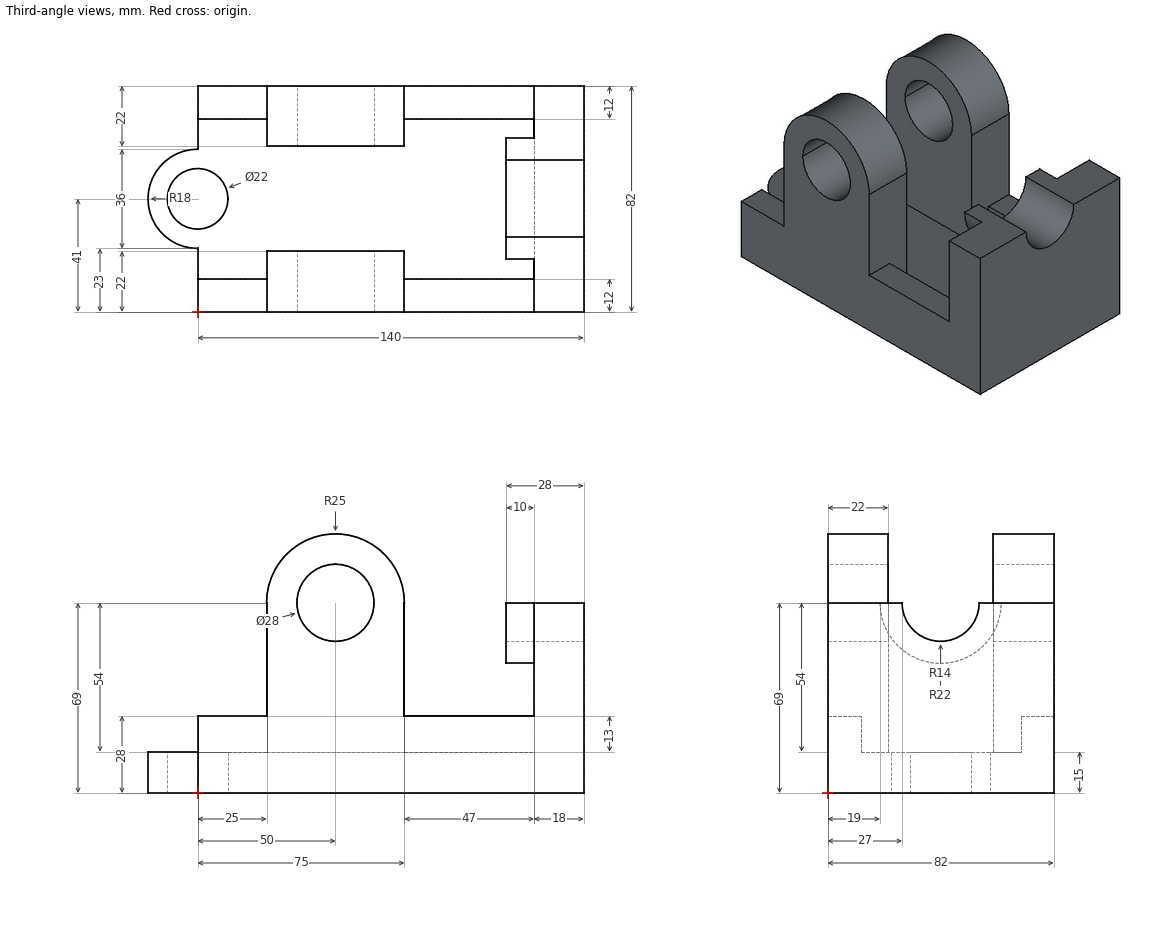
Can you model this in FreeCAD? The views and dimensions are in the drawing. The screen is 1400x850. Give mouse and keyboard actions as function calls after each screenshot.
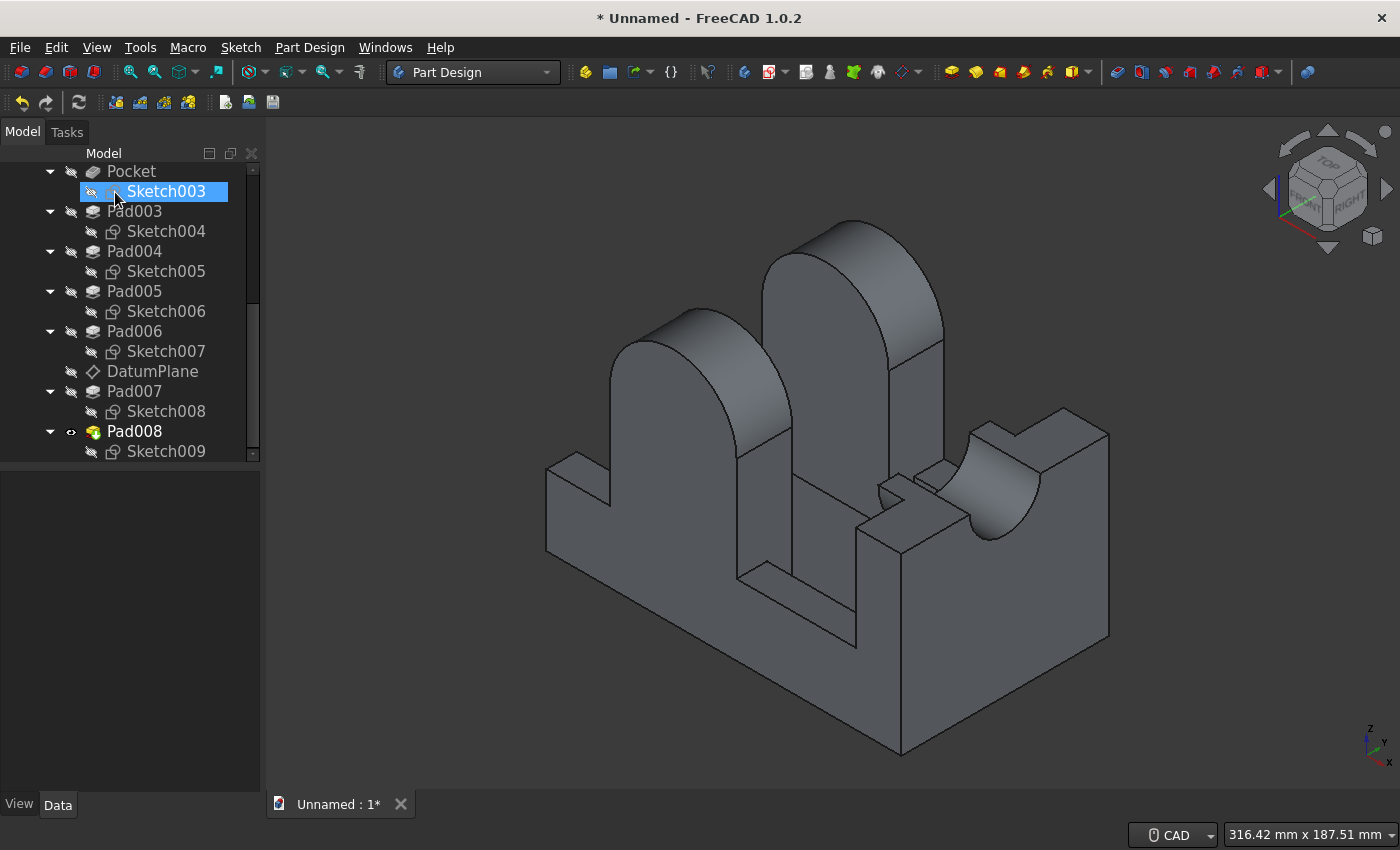
click(805, 535)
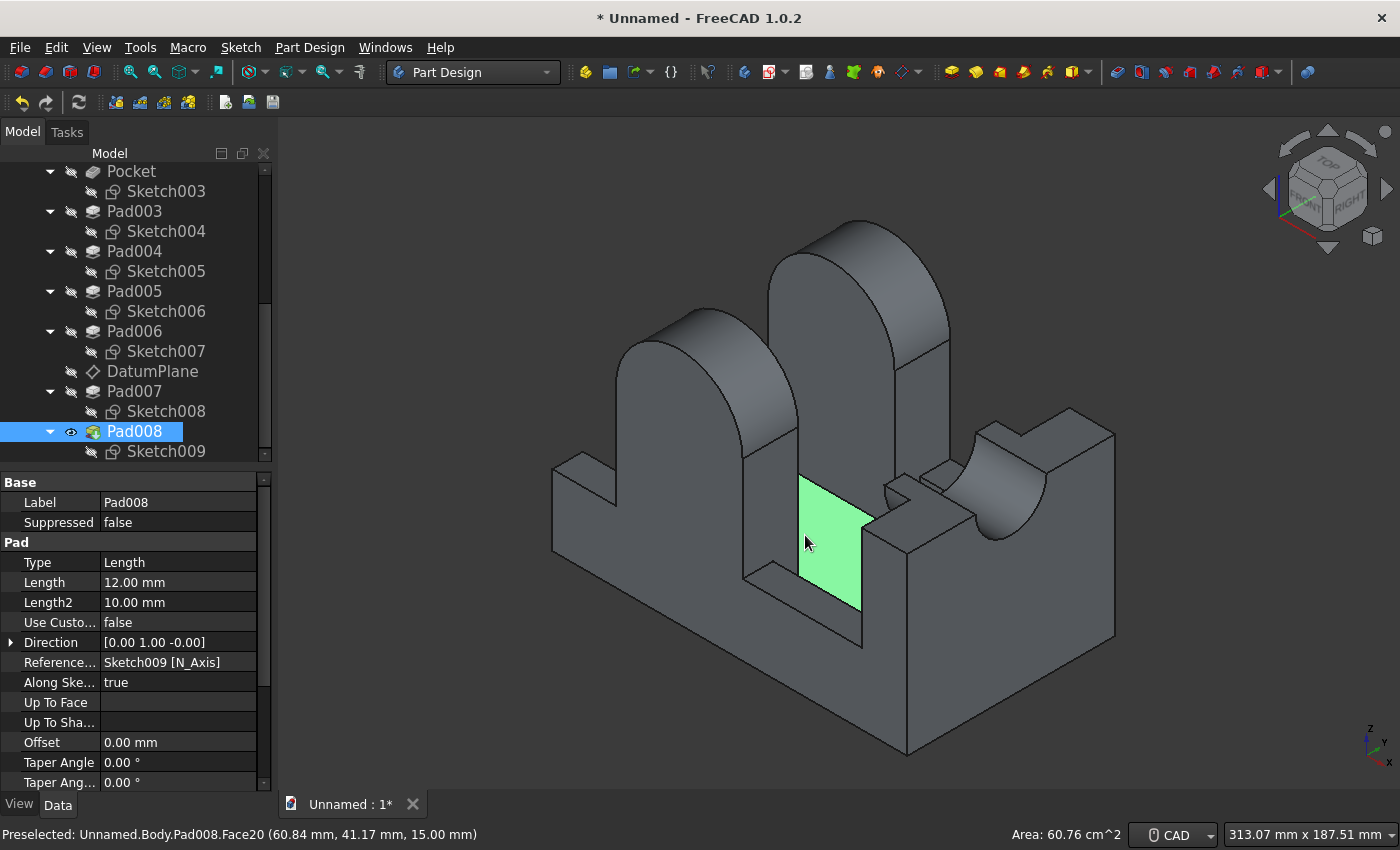
click(770, 72)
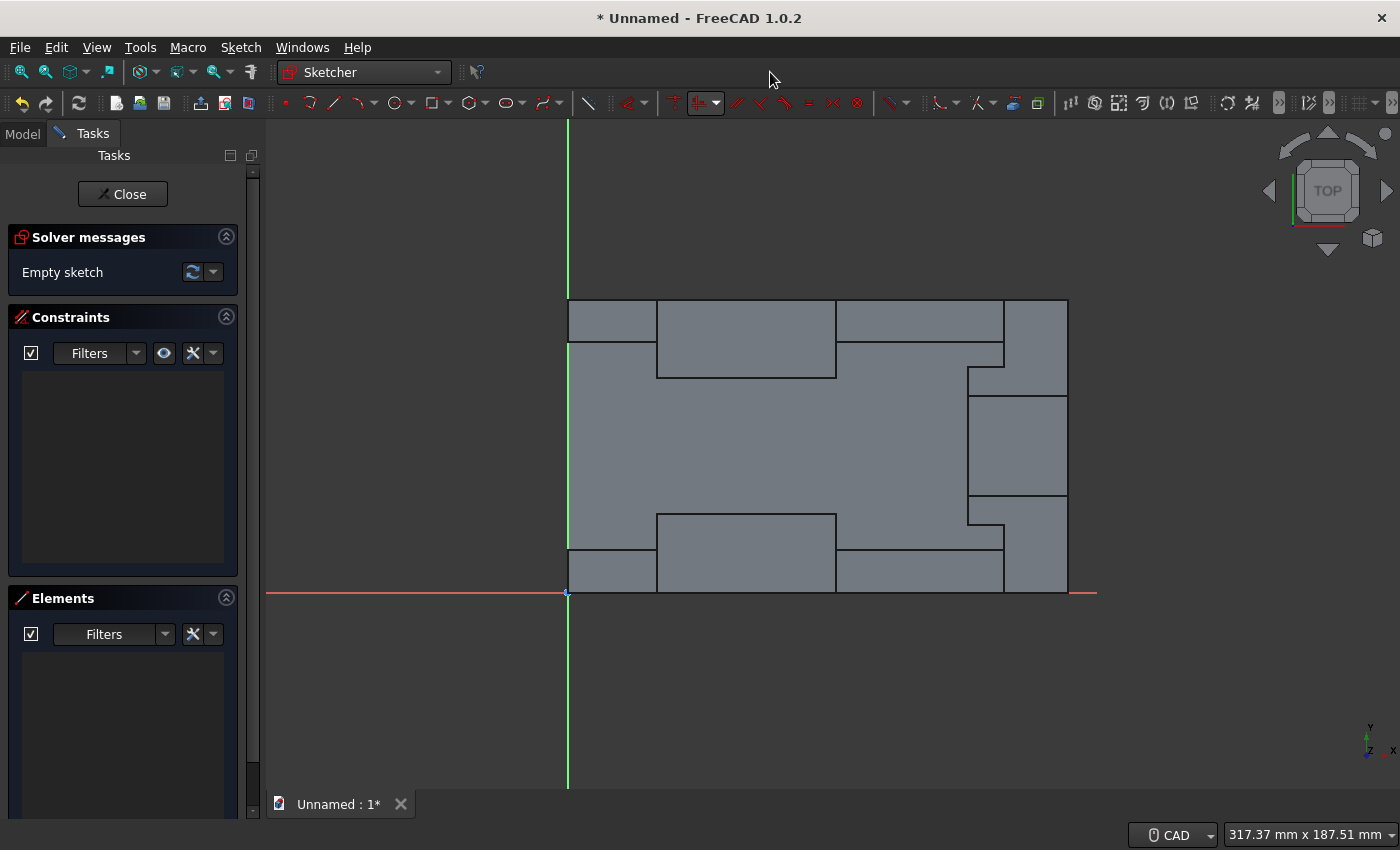
scroll(349, 514, up, 4)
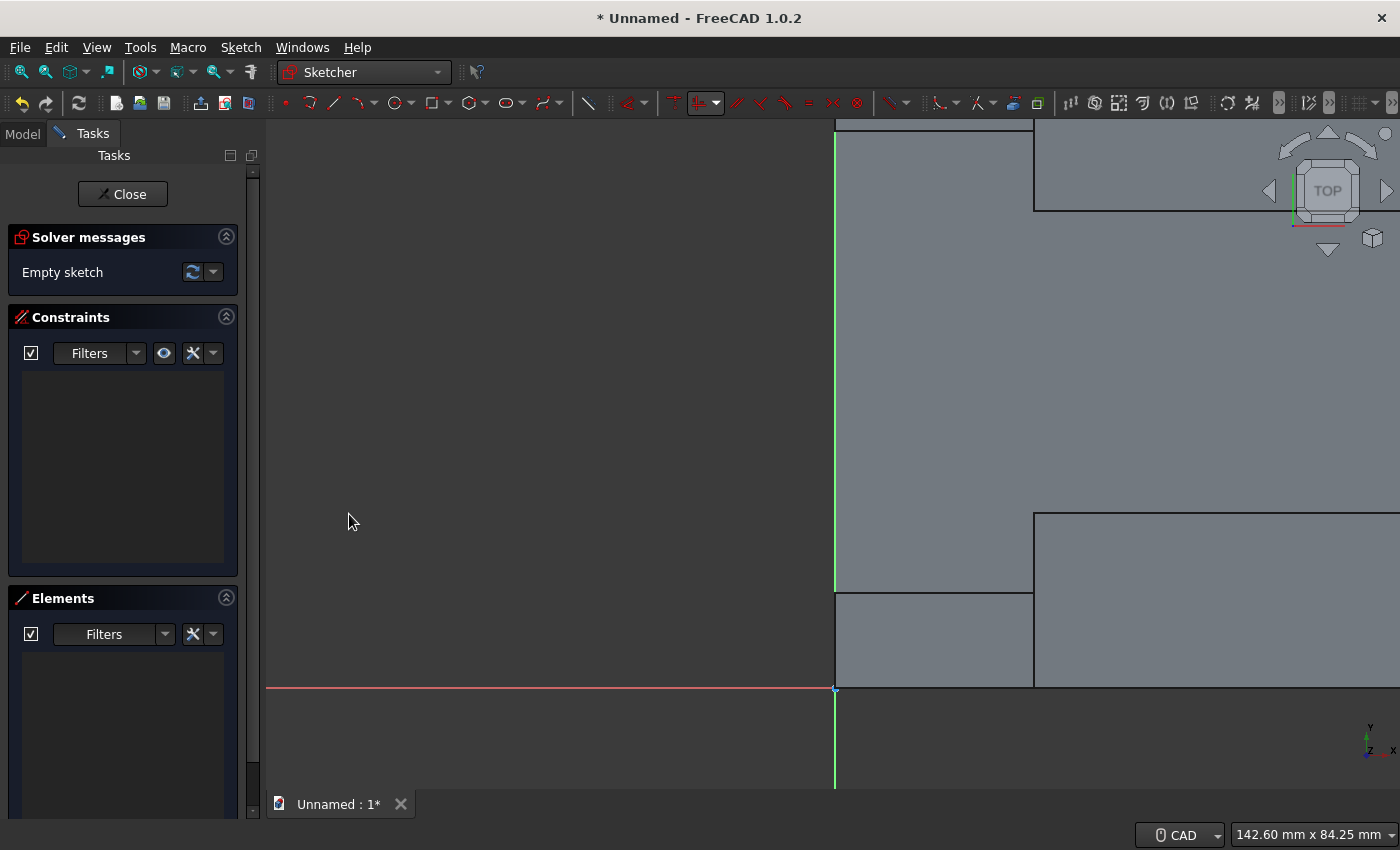
click(334, 104)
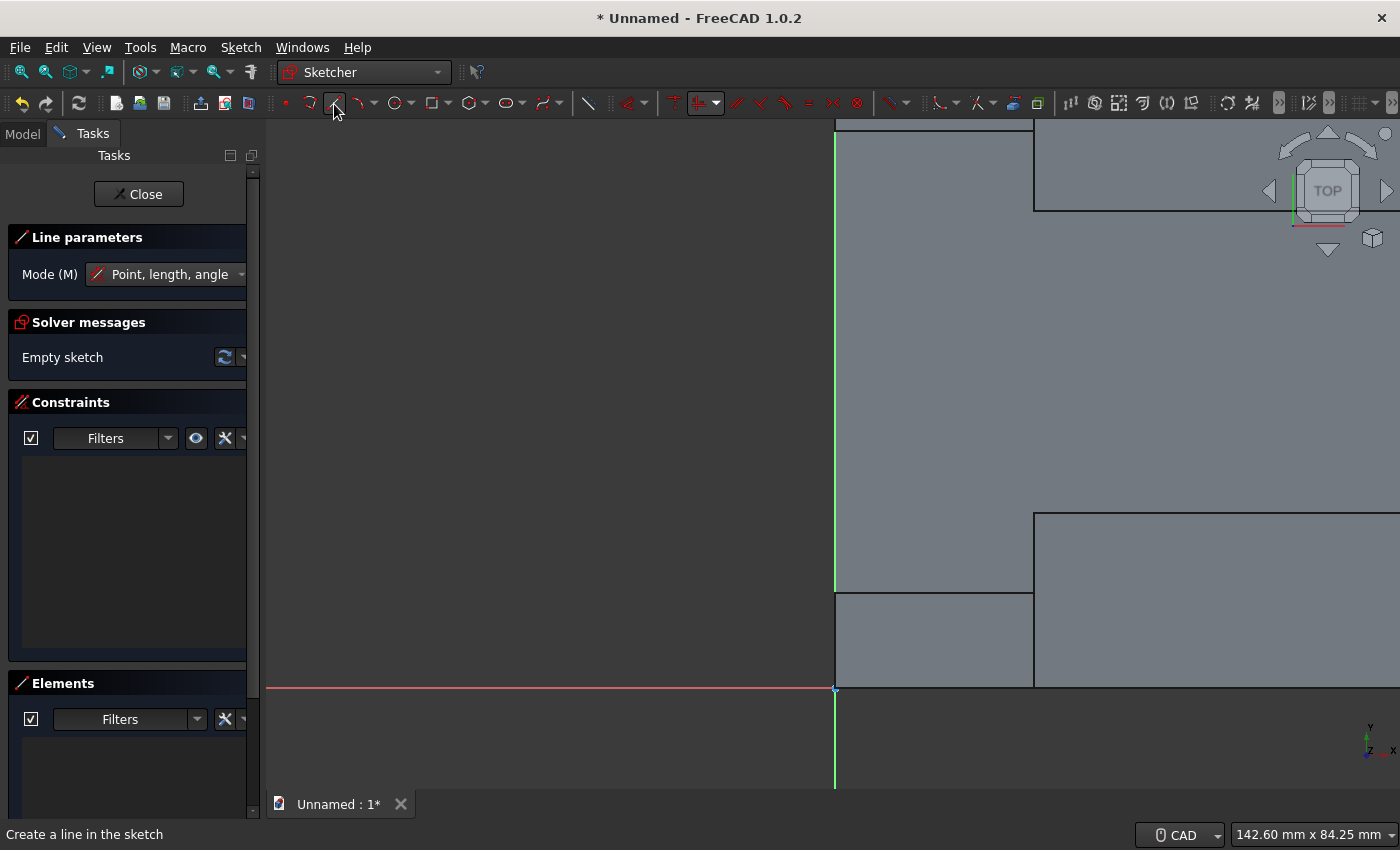
click(835, 505)
click(826, 219)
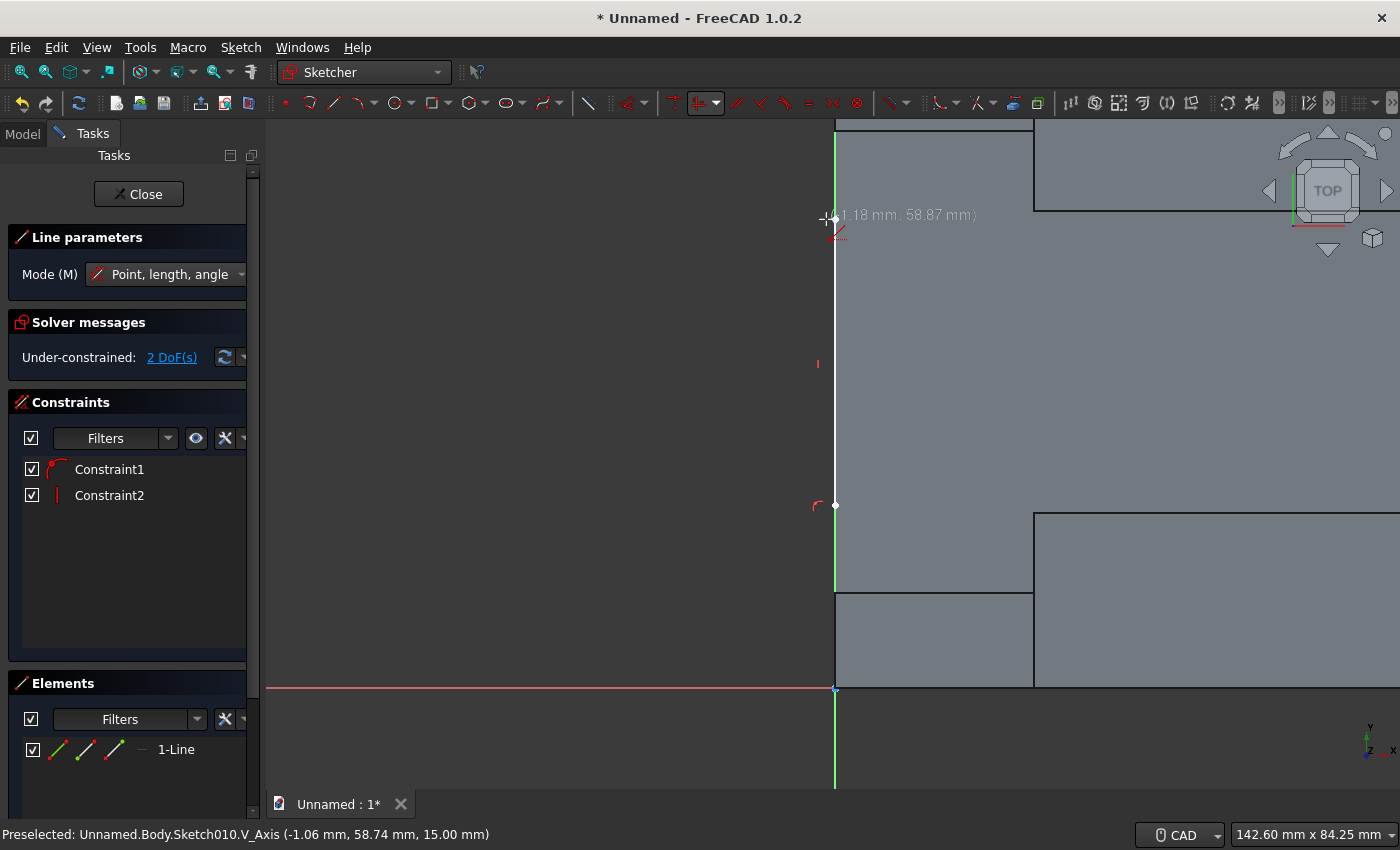
click(358, 104)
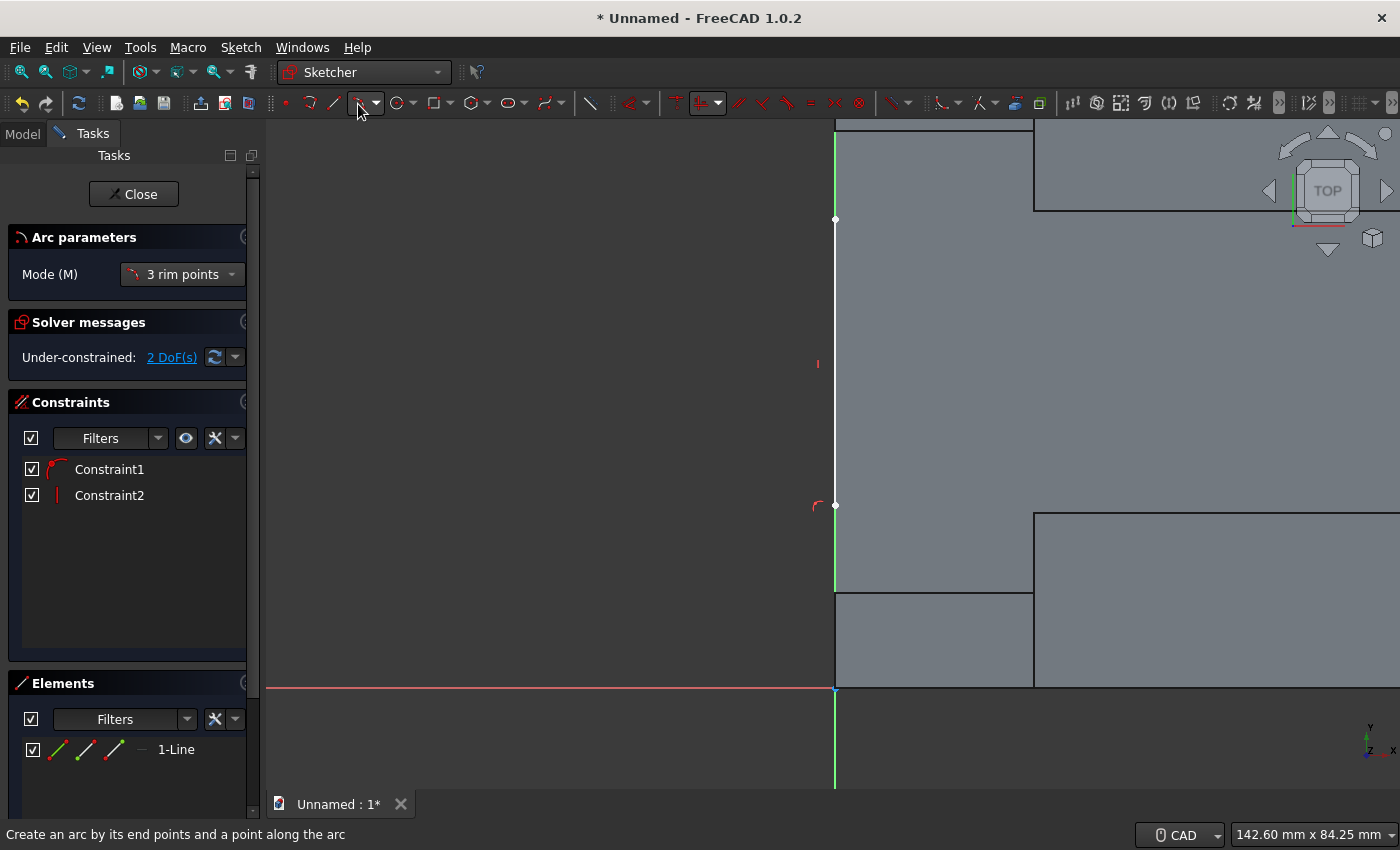
click(826, 219)
click(835, 506)
click(692, 362)
key(Escape)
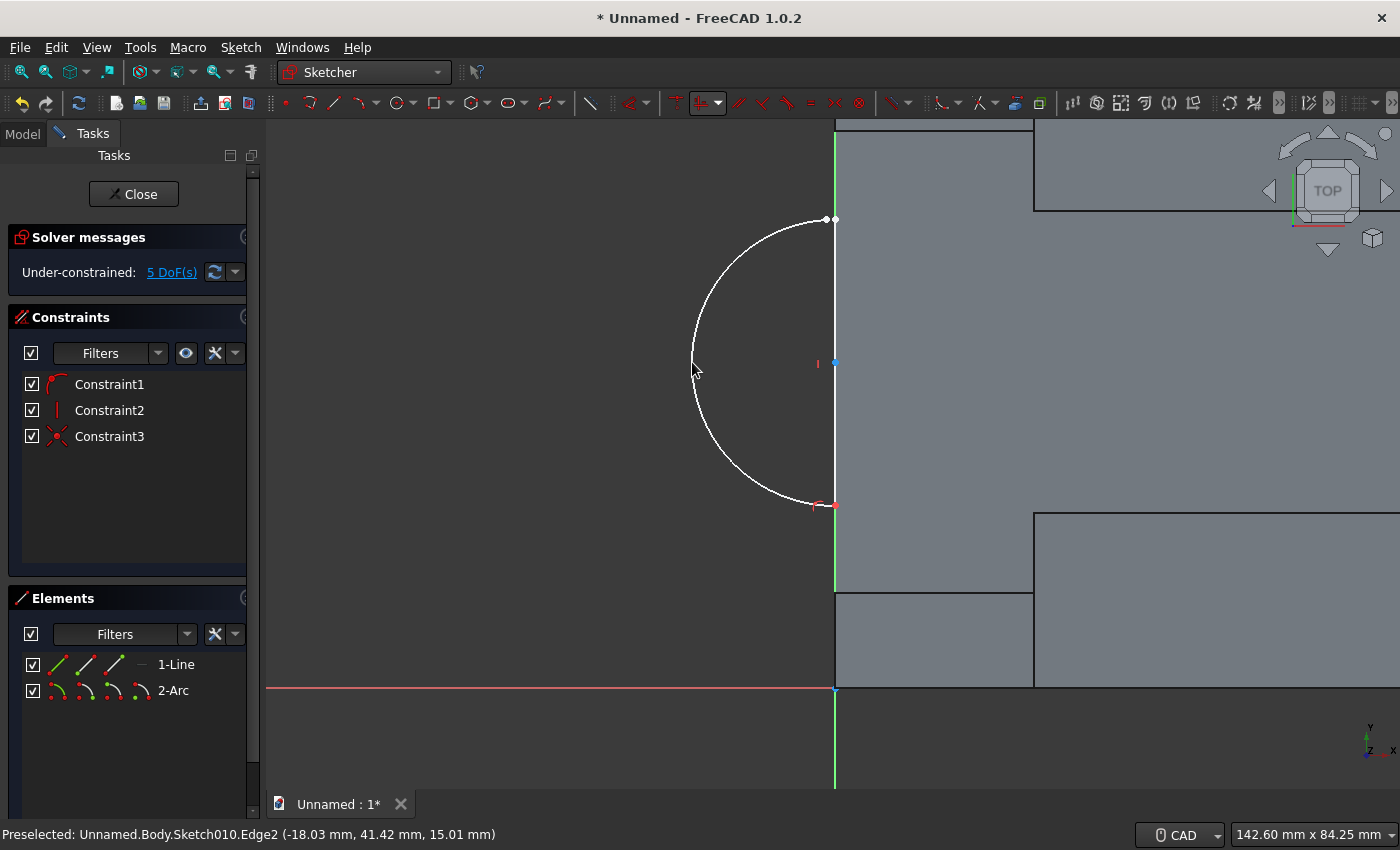
click(835, 363)